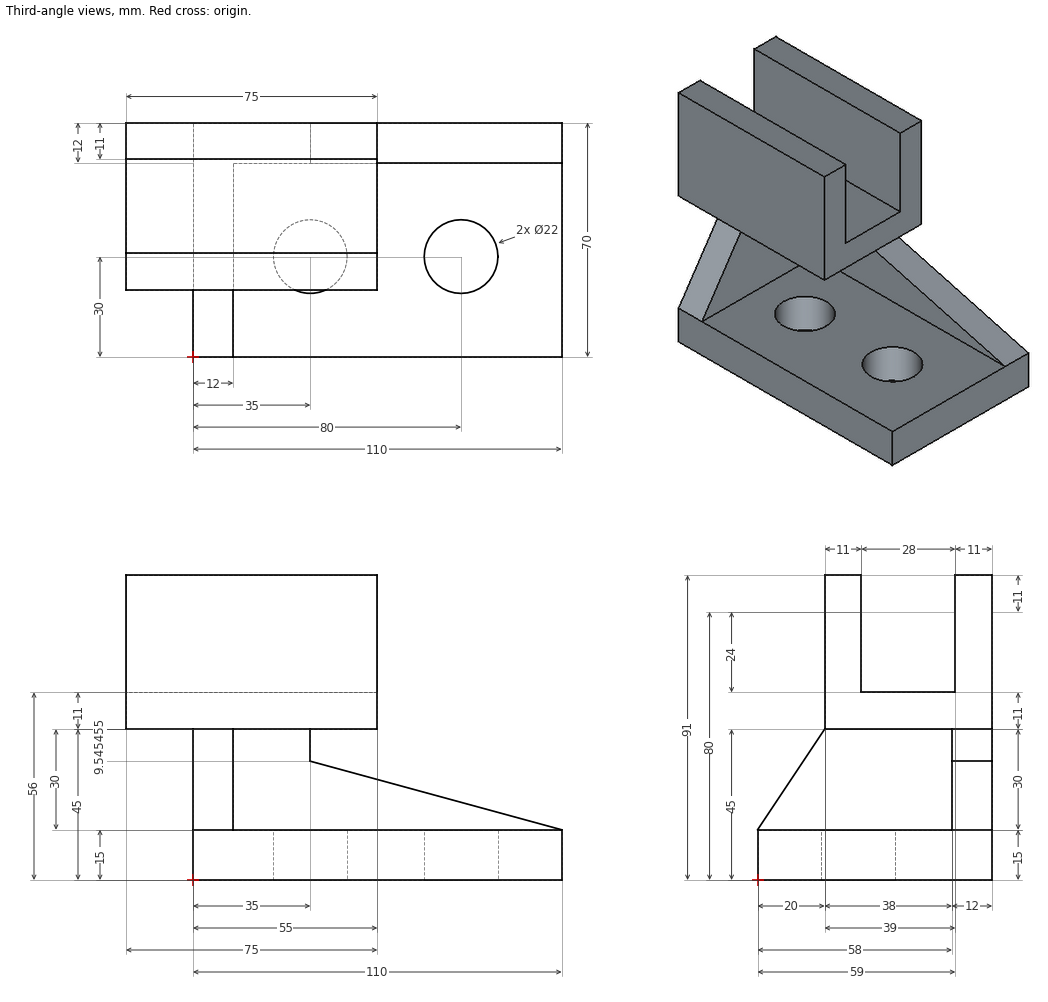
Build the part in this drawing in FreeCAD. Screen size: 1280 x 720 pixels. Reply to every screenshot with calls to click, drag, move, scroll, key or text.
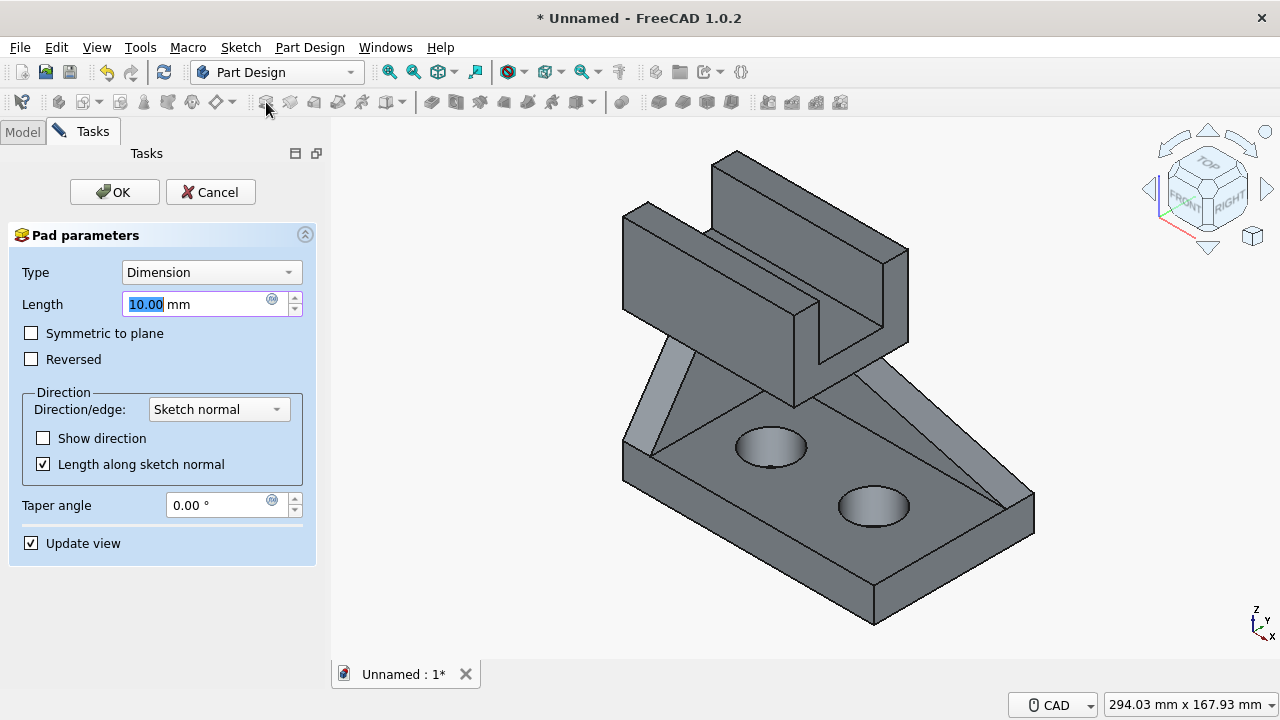
text(75)
key(Tab)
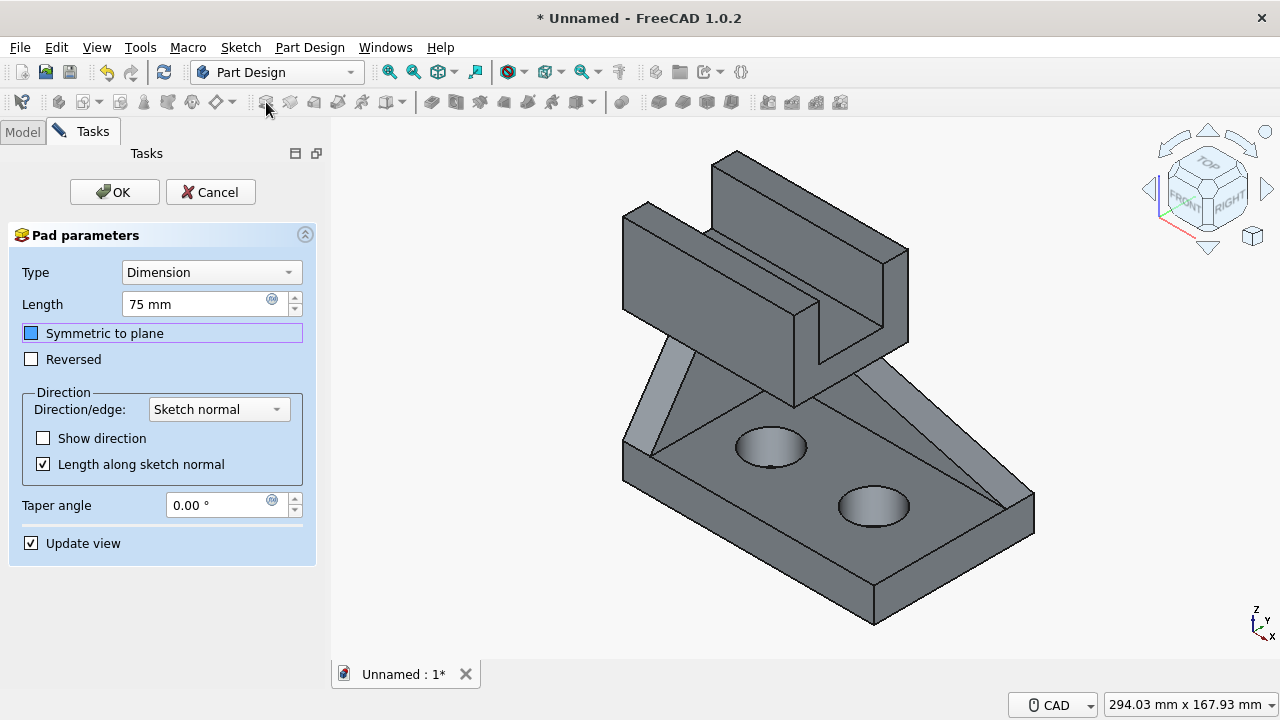
click(30, 359)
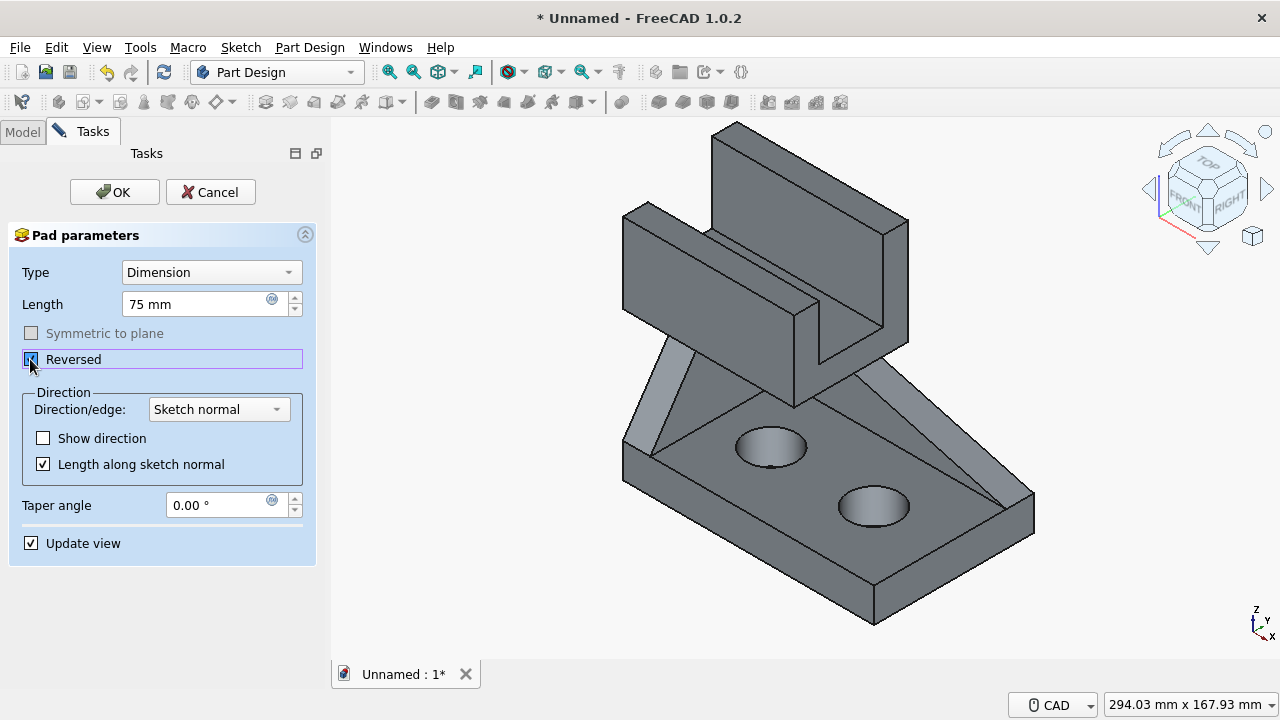
click(115, 192)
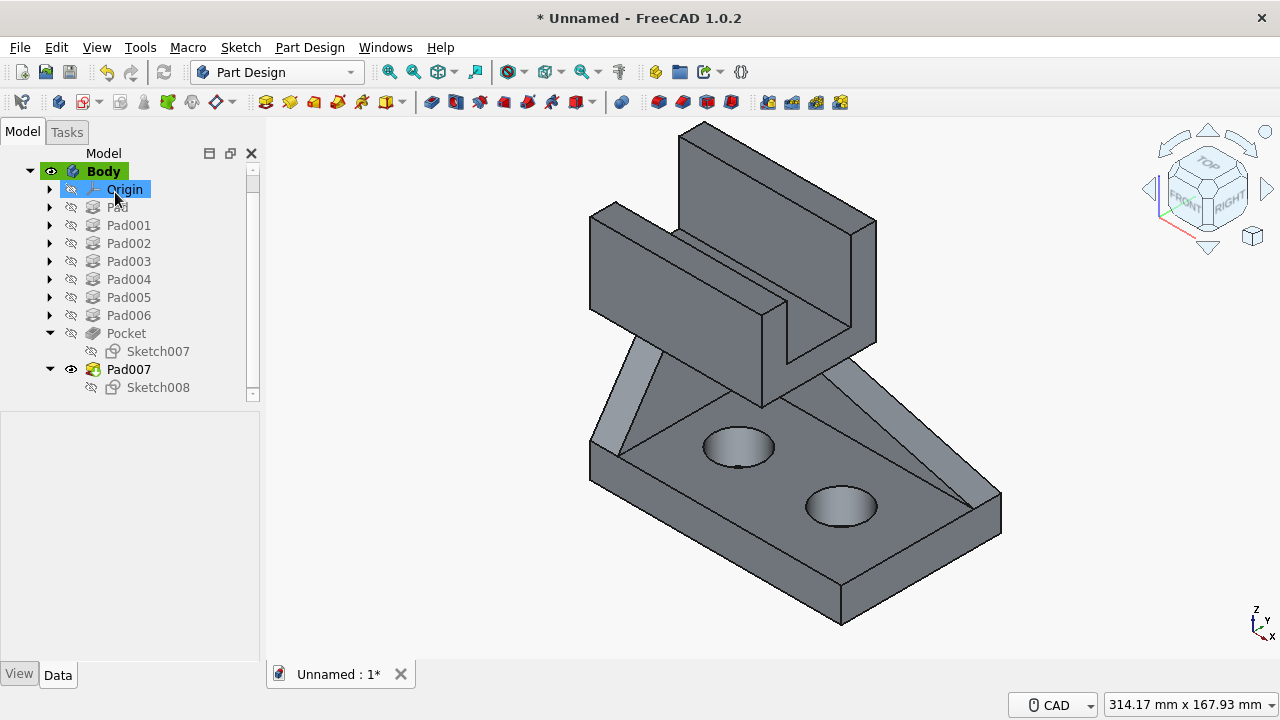
click(770, 324)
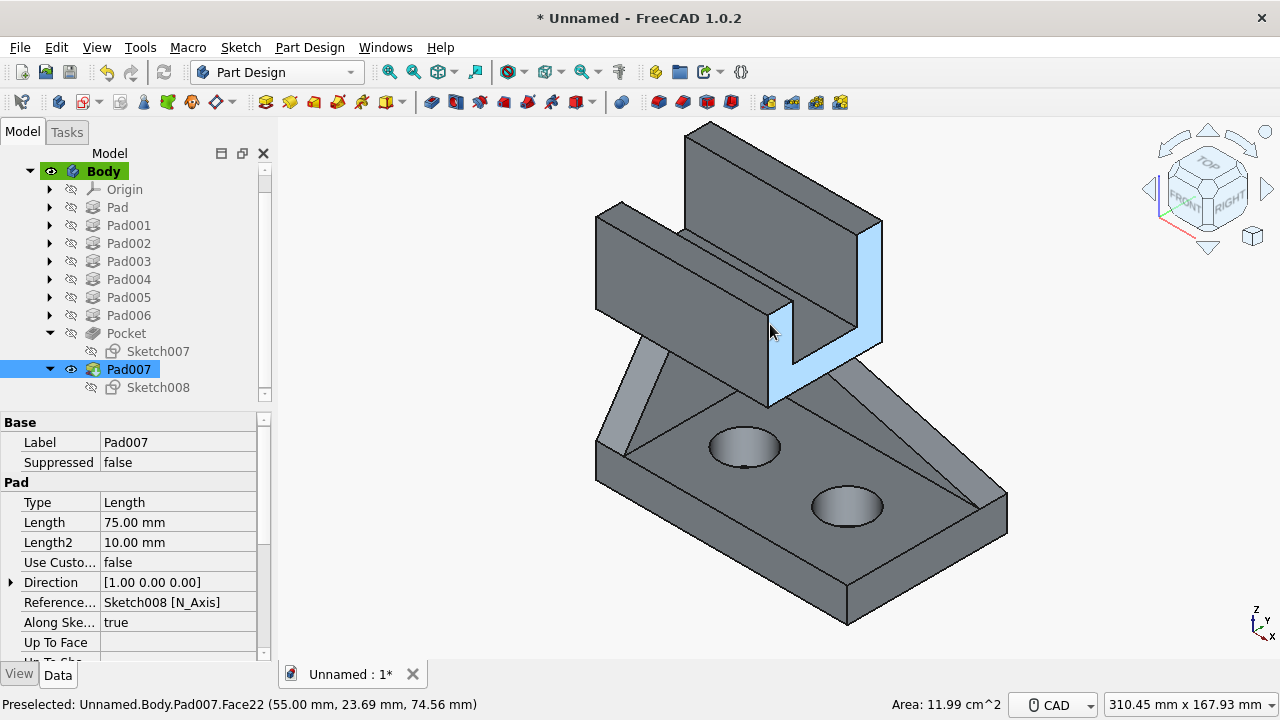
click(84, 102)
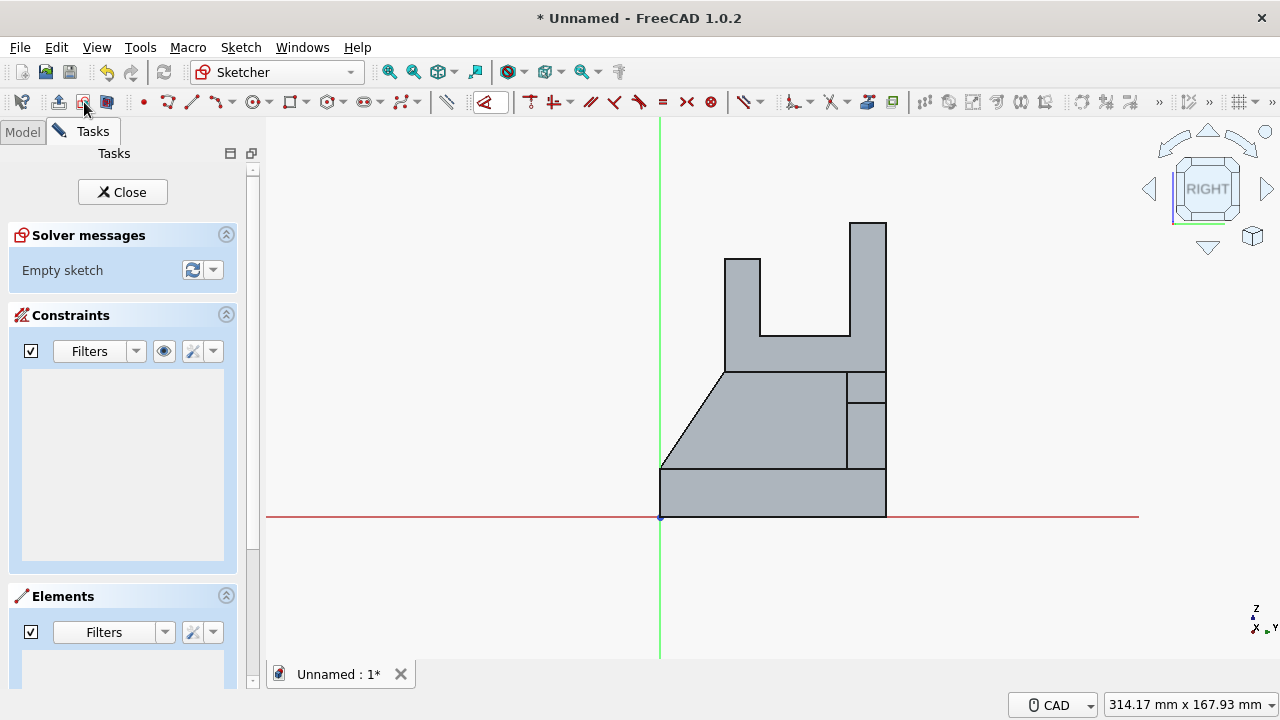
click(108, 102)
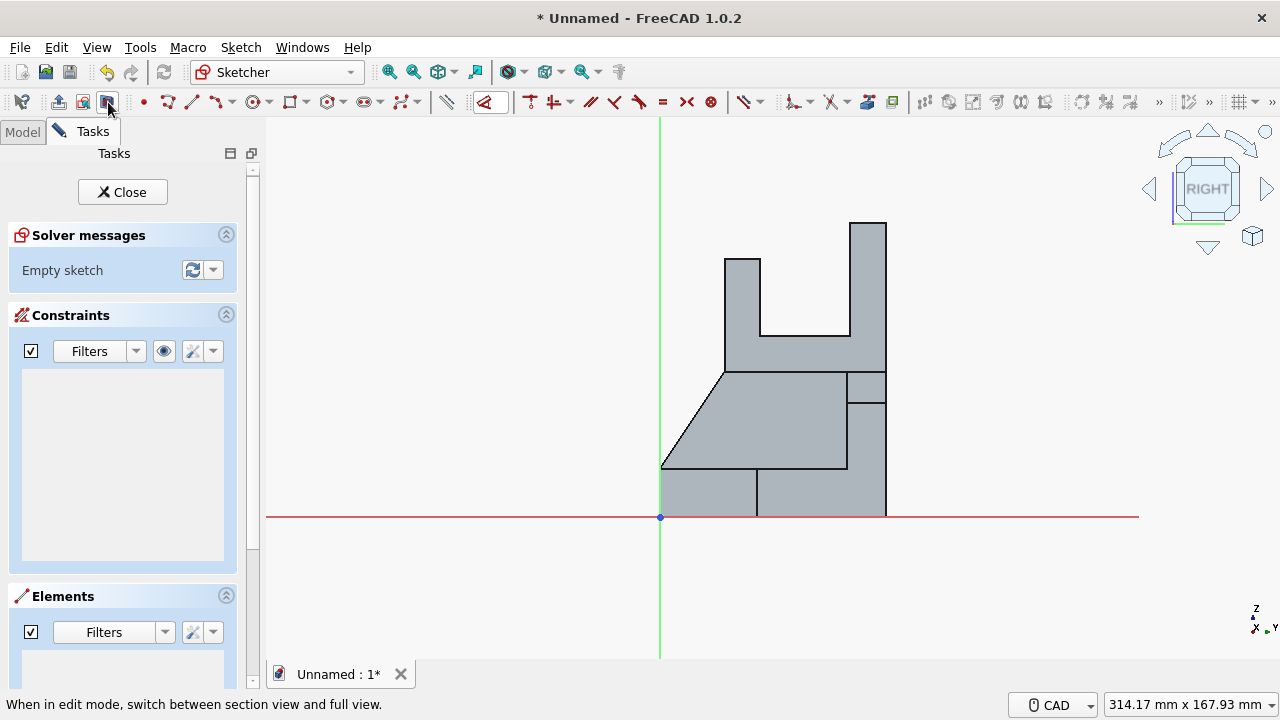
scroll(747, 223, up, 11)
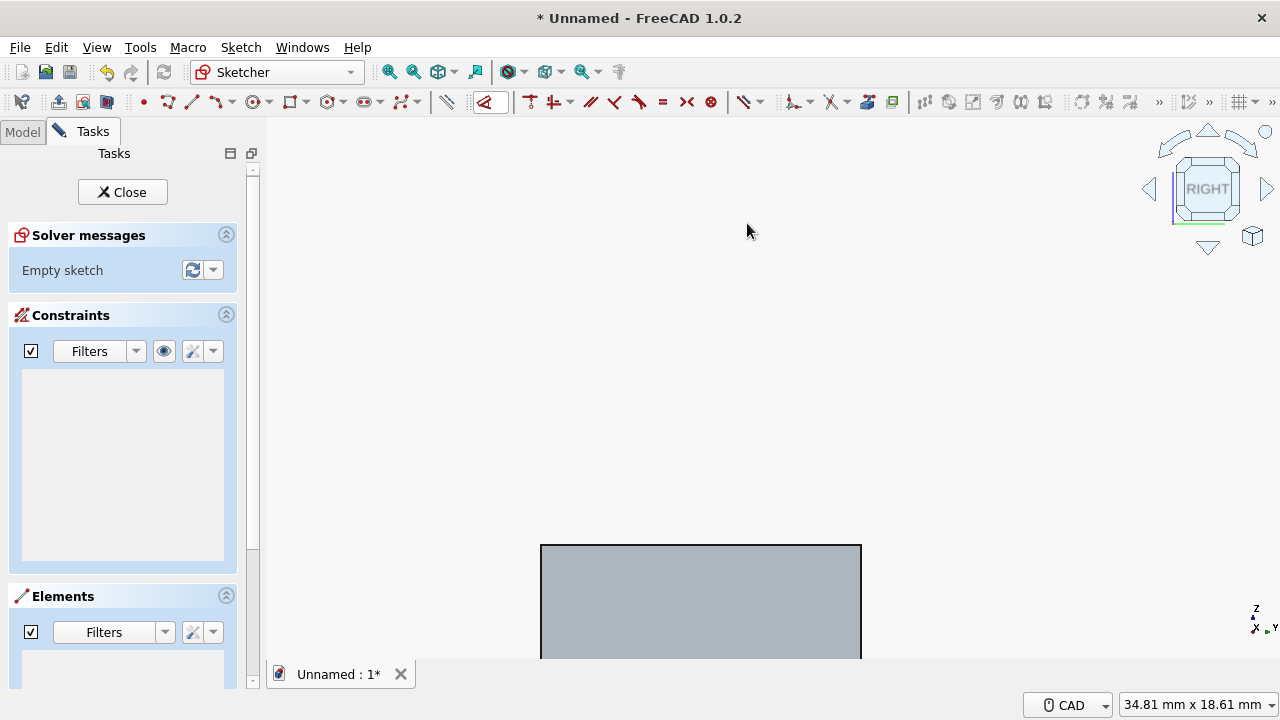
key(g)
key(r)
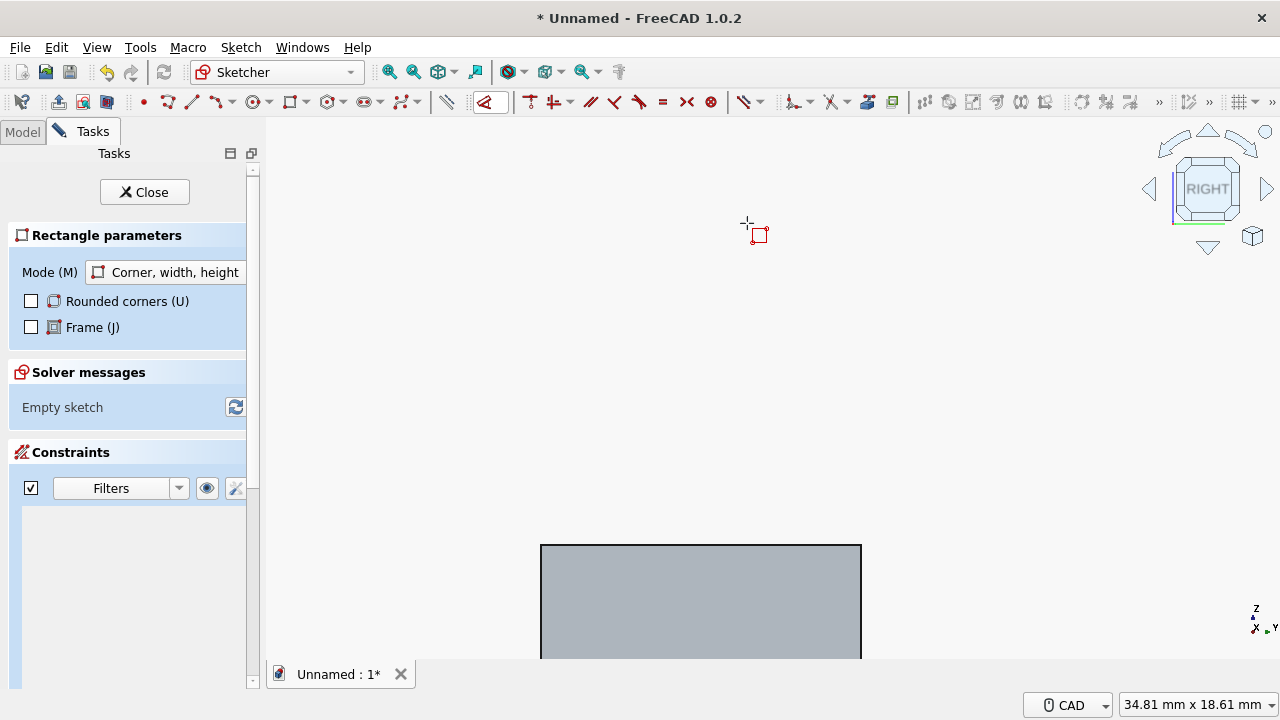
click(541, 225)
move(861, 545)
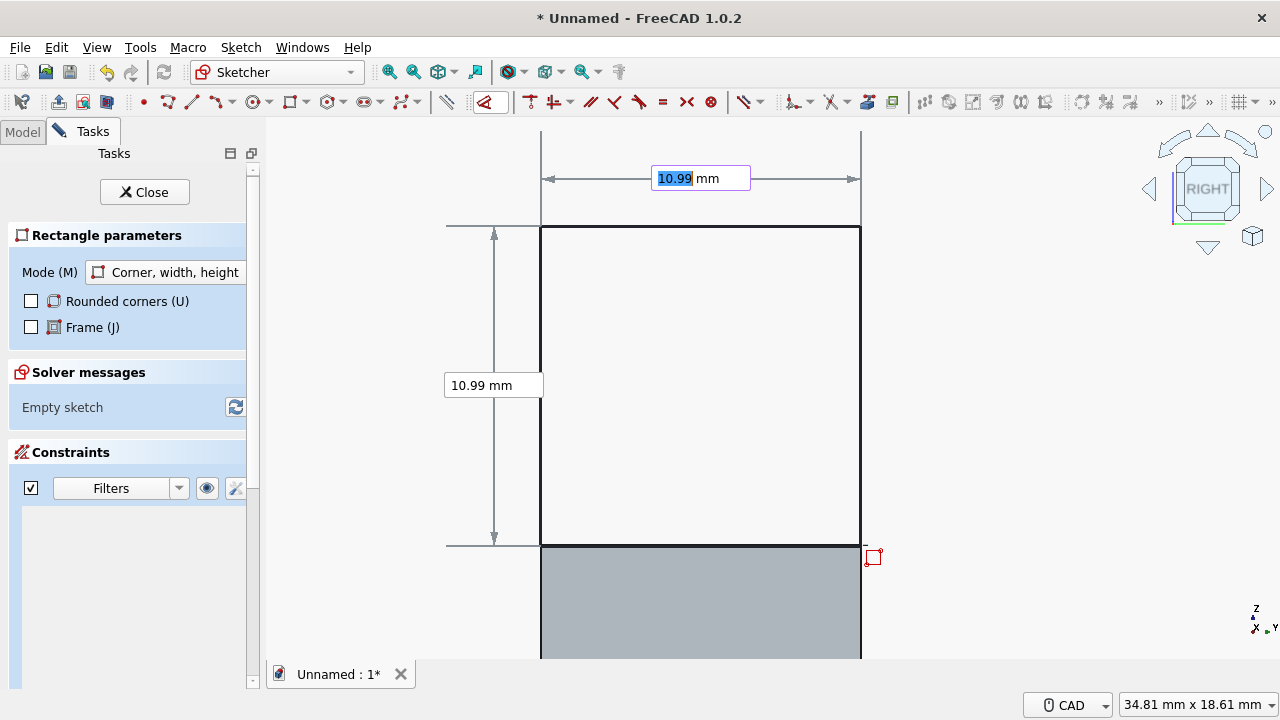
text(11)
key(Tab)
text(11)
key(Return)
key(Escape)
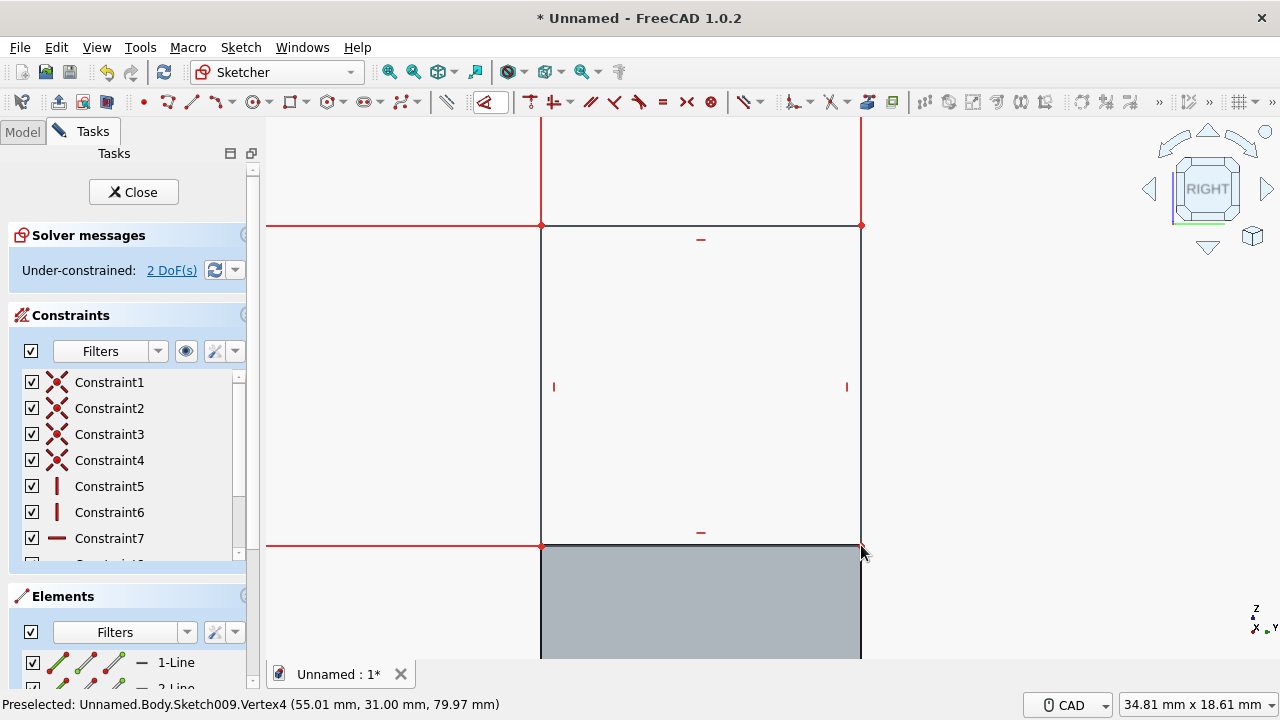
click(541, 226)